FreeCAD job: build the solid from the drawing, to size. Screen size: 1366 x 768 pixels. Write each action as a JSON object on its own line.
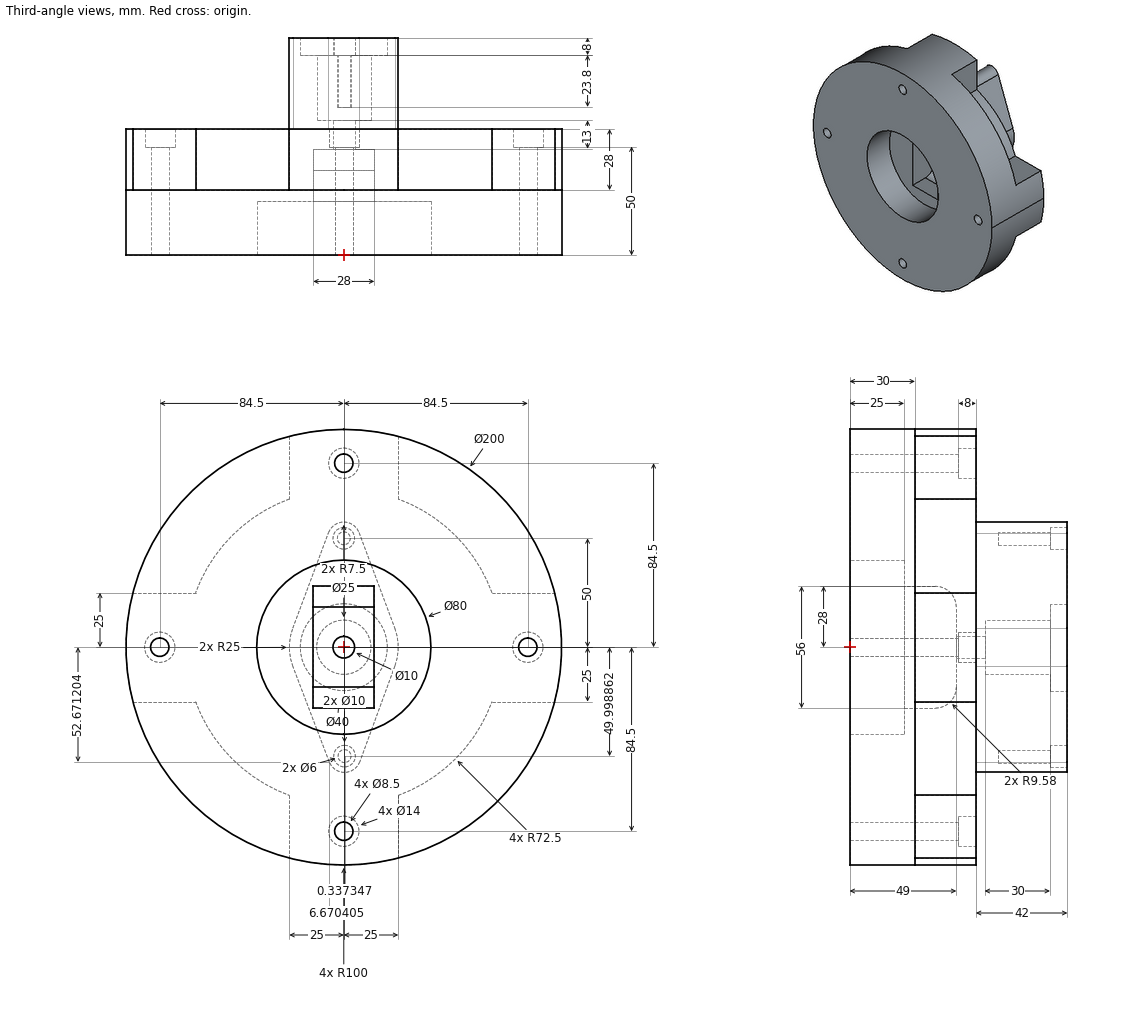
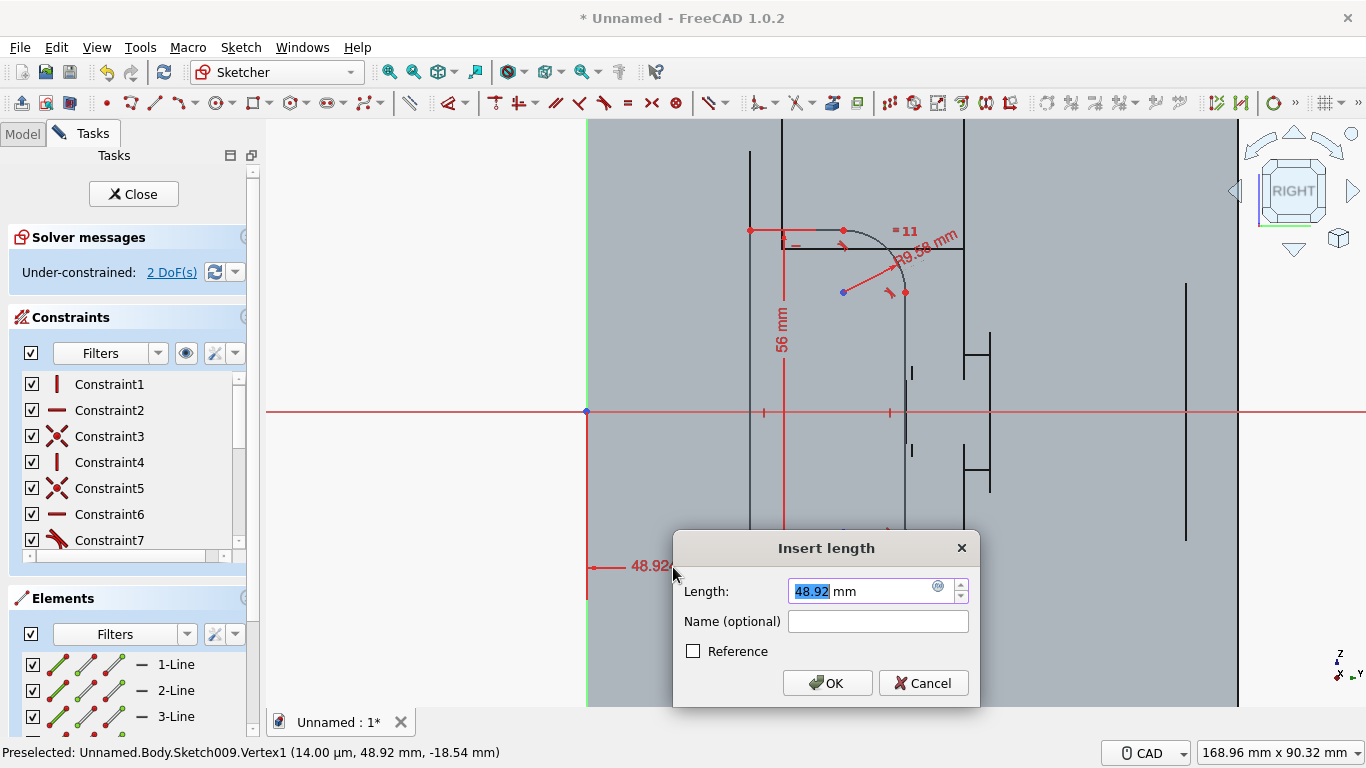
{"action": "type", "text": "49"}
{"action": "key", "text": "Return"}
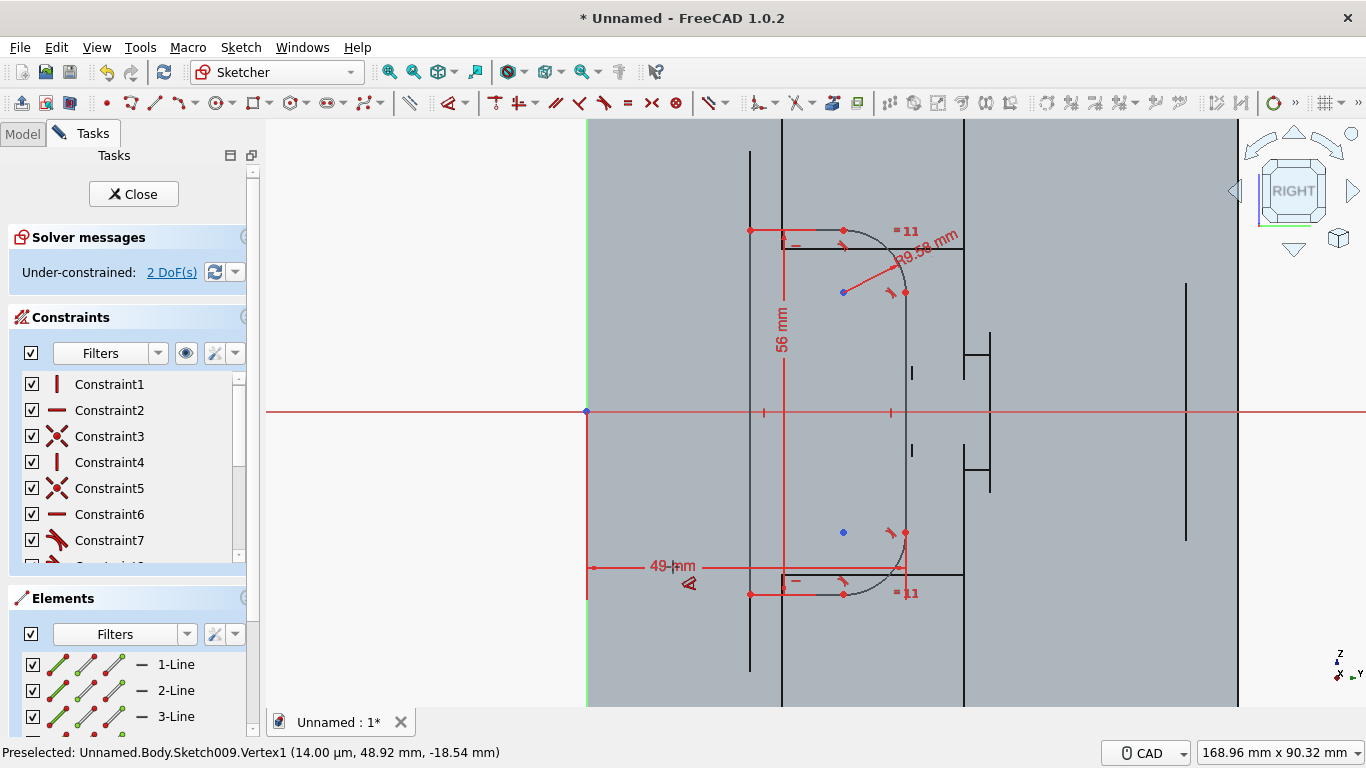
{"action": "left_click", "coordinate": [843, 230]}
{"action": "left_click", "coordinate": [553, 321]}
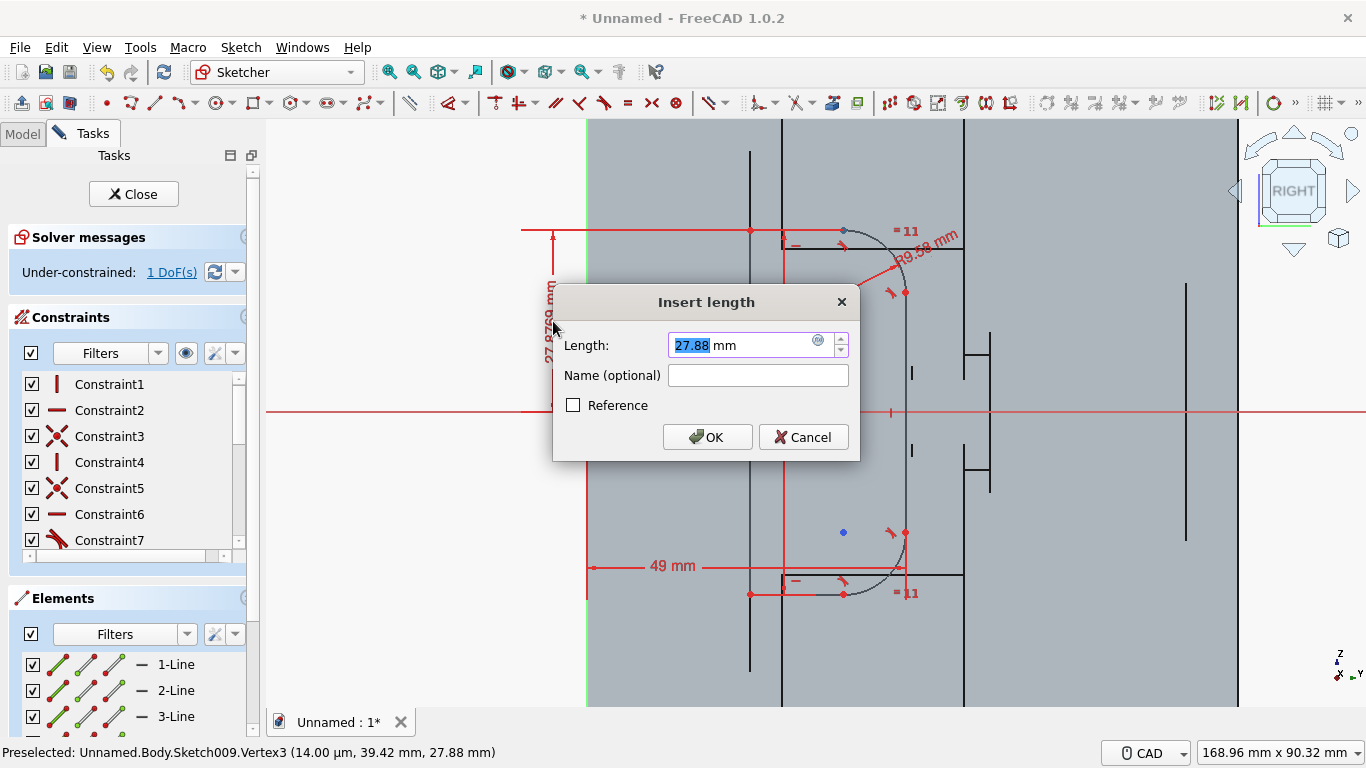
{"action": "type", "text": "28"}
{"action": "key", "text": "Return"}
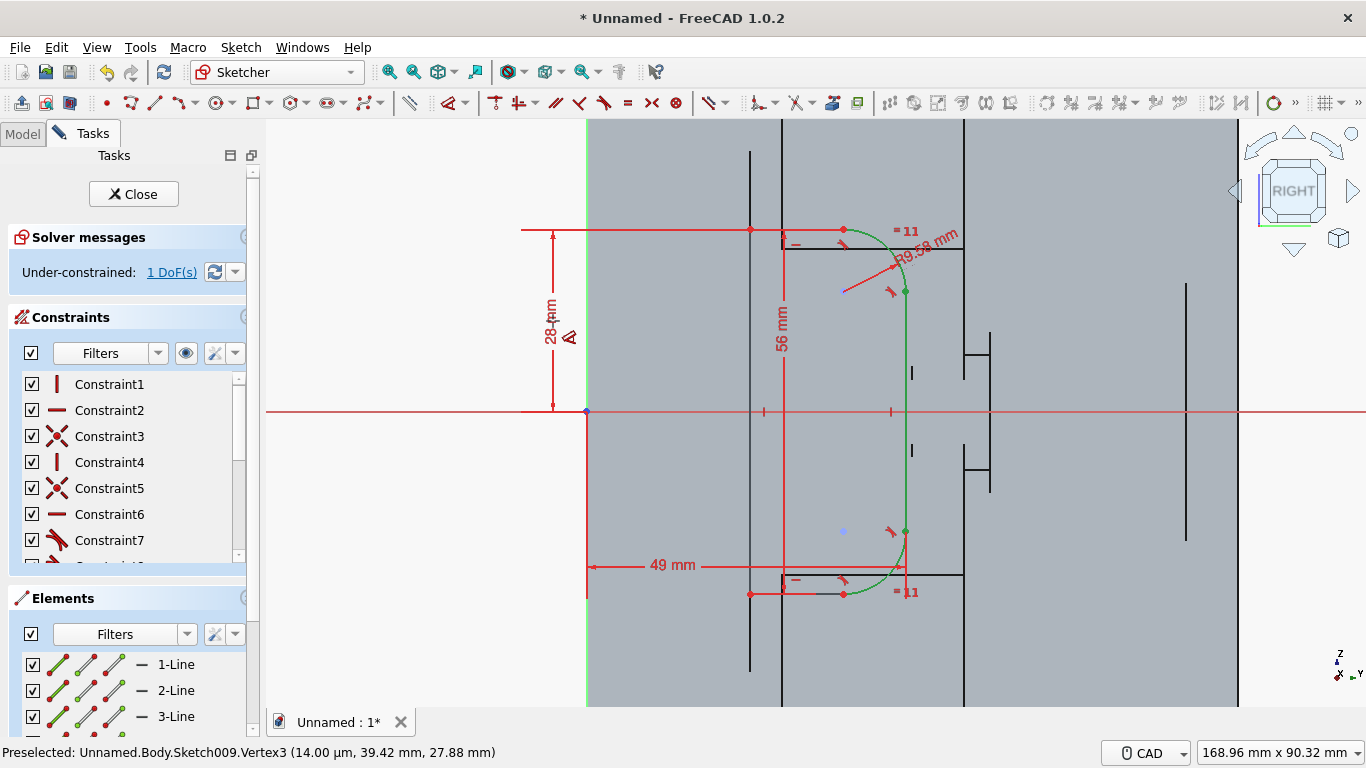
{"action": "left_click", "coordinate": [750, 230]}
{"action": "left_click", "coordinate": [668, 196]}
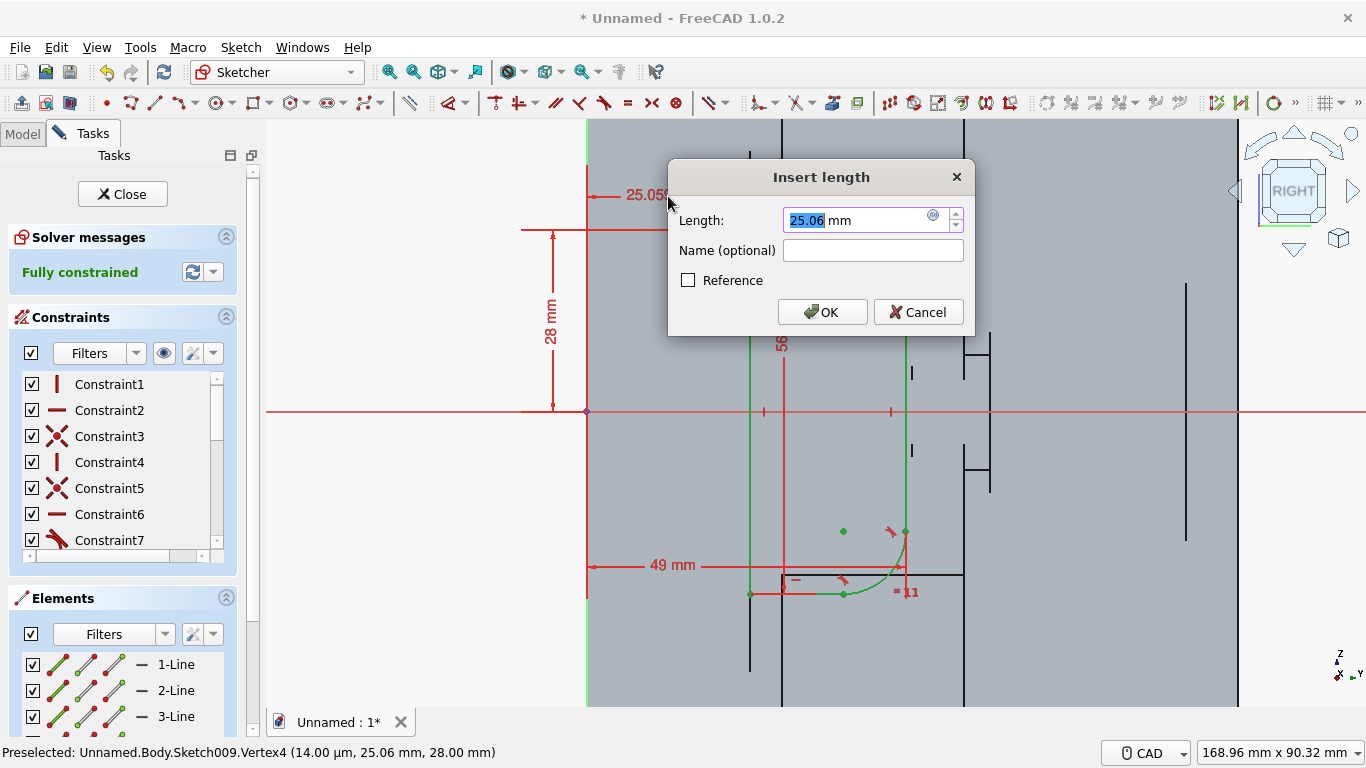
{"action": "type", "text": "25"}
{"action": "key", "text": "Return"}
{"action": "key", "text": "Escape"}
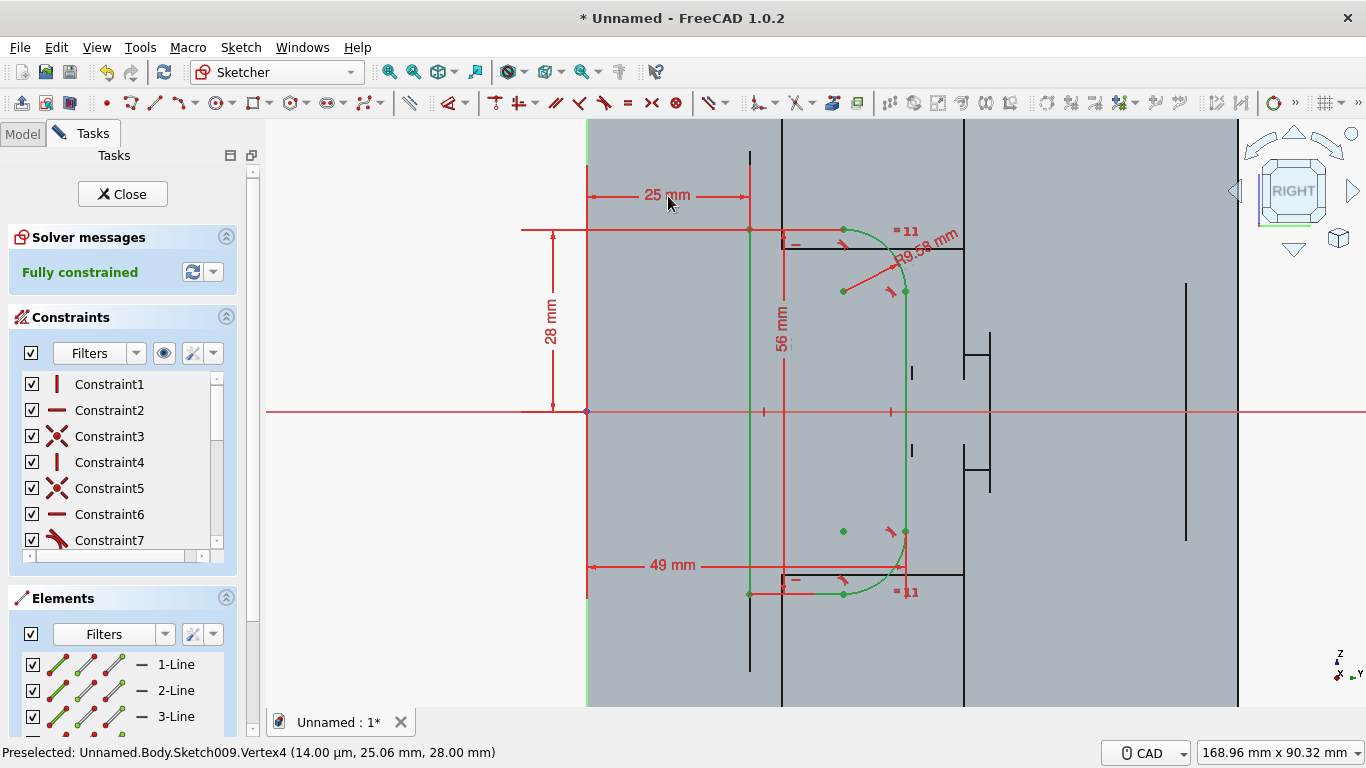
{"action": "left_click", "coordinate": [123, 194]}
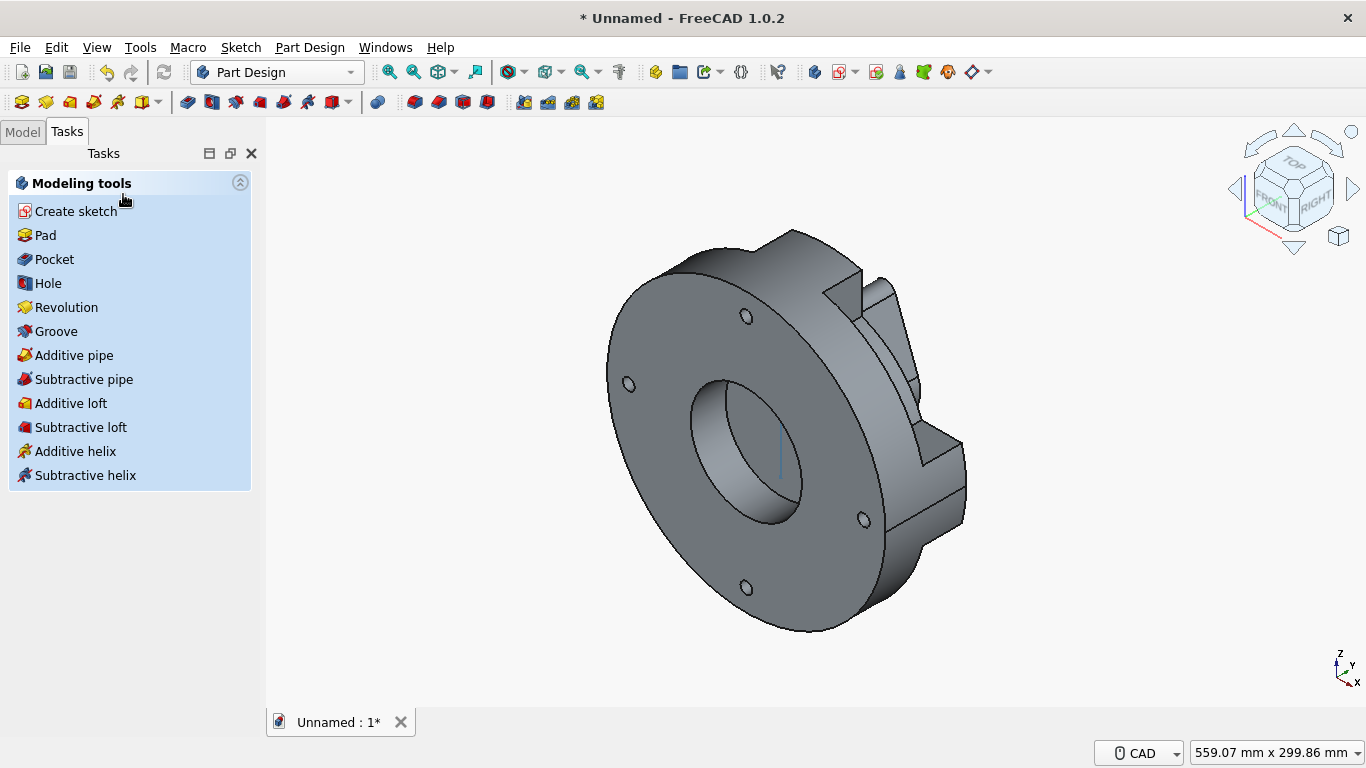
{"action": "left_click", "coordinate": [188, 102]}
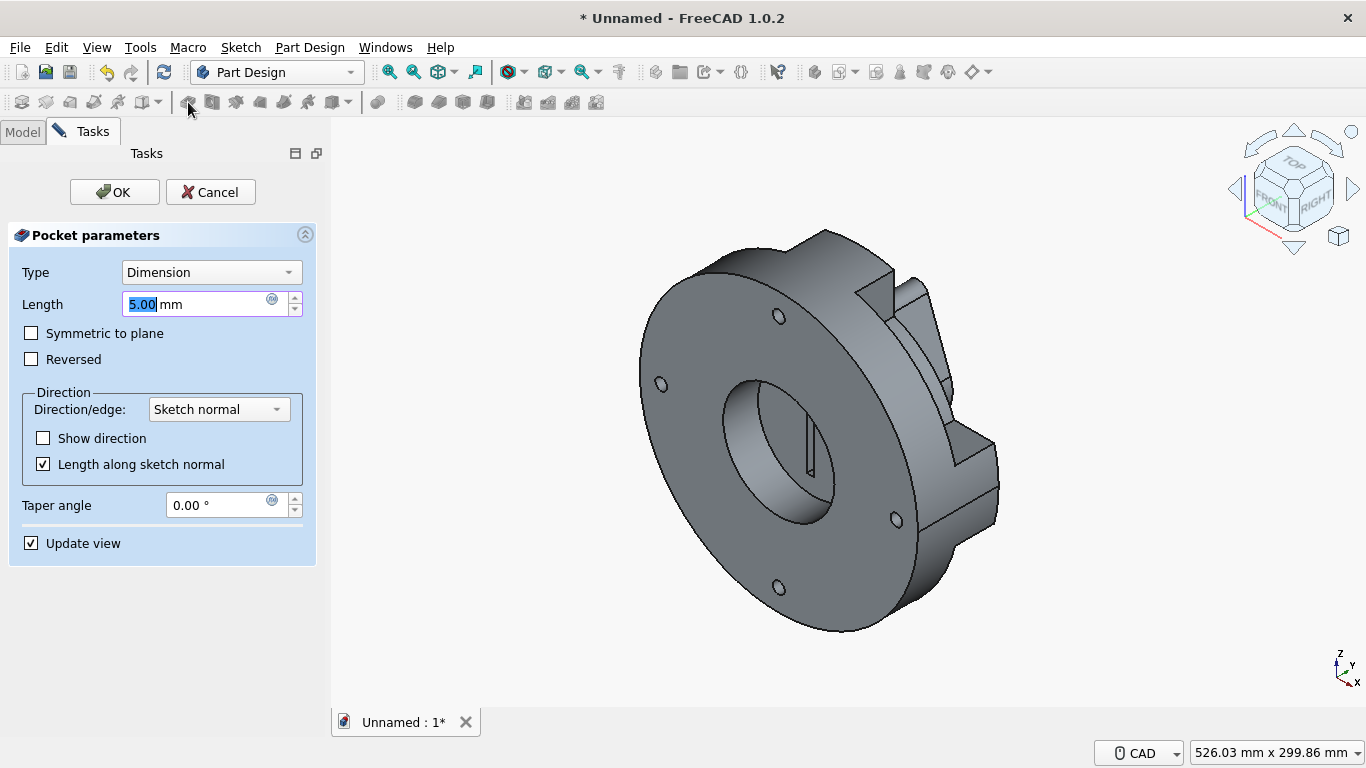
{"action": "type", "text": "28"}
{"action": "key", "text": "Tab"}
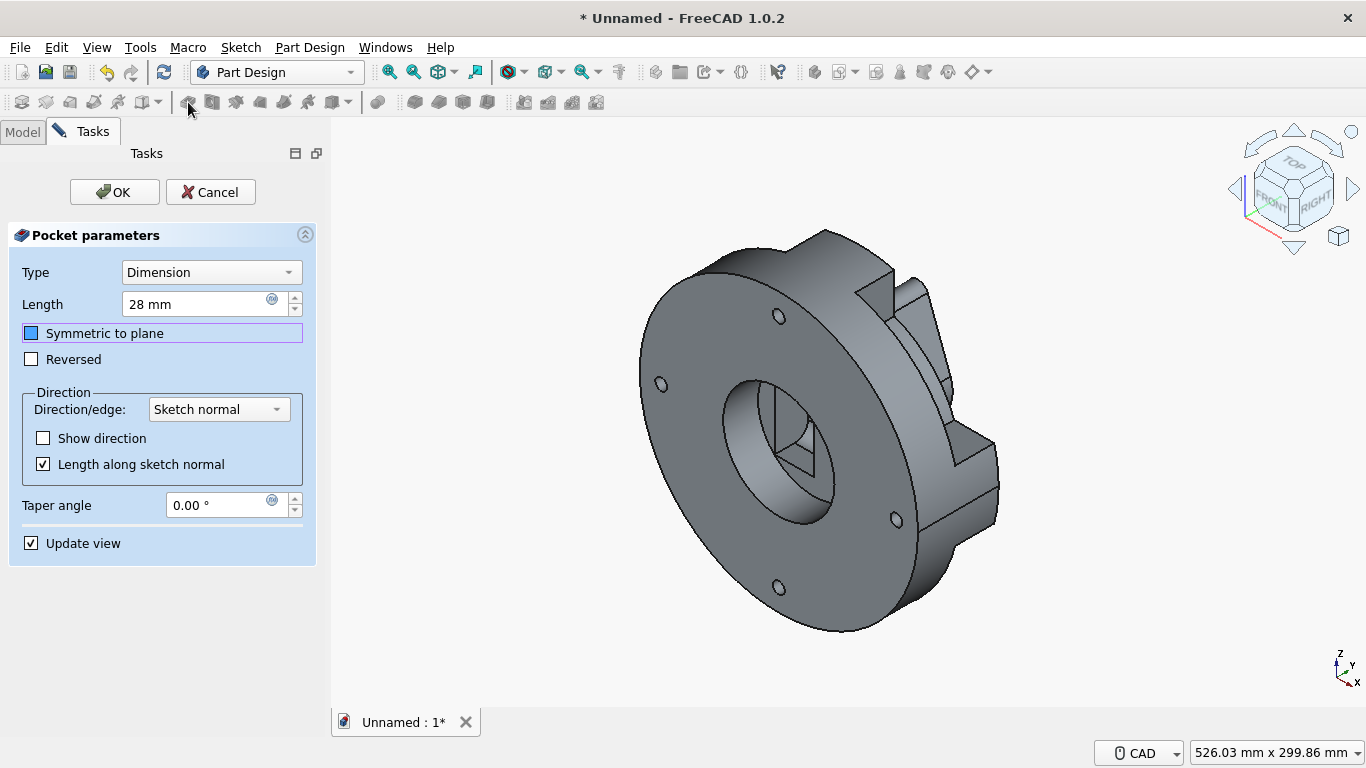
{"action": "left_click", "coordinate": [30, 333]}